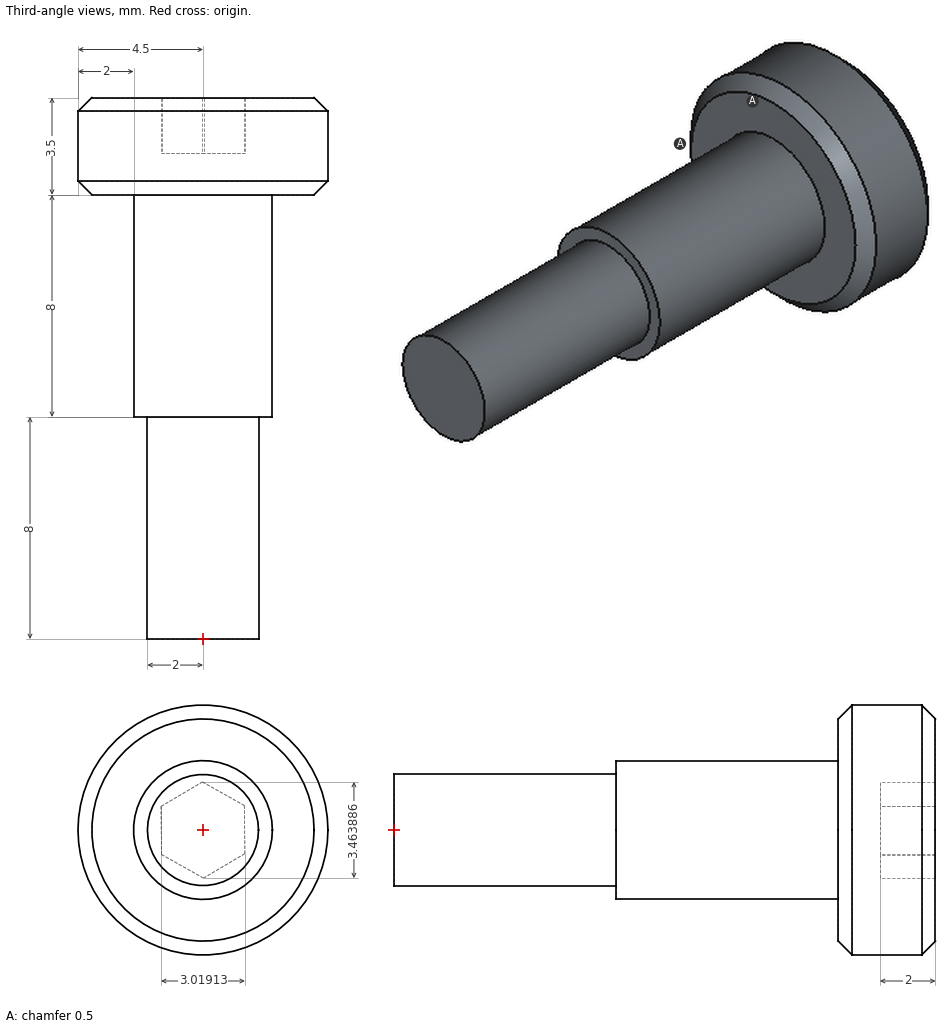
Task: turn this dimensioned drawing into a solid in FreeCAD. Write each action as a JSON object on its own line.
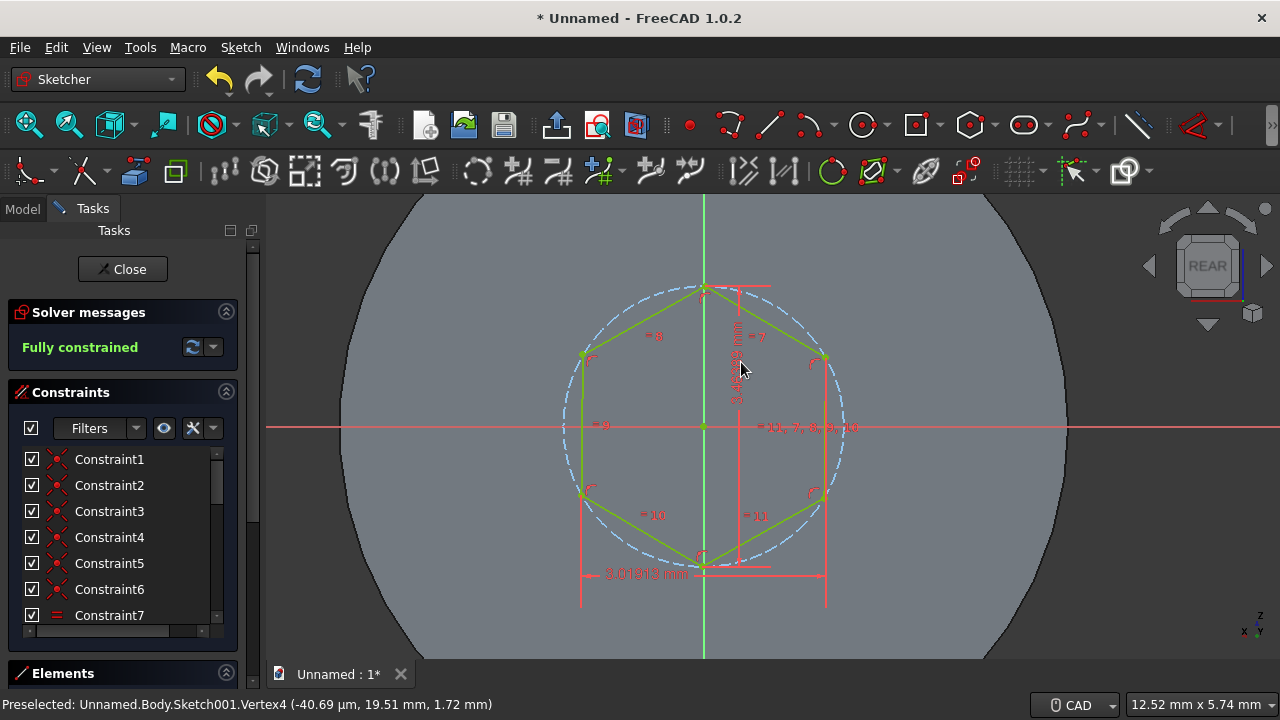
{"action": "left_click", "coordinate": [123, 269]}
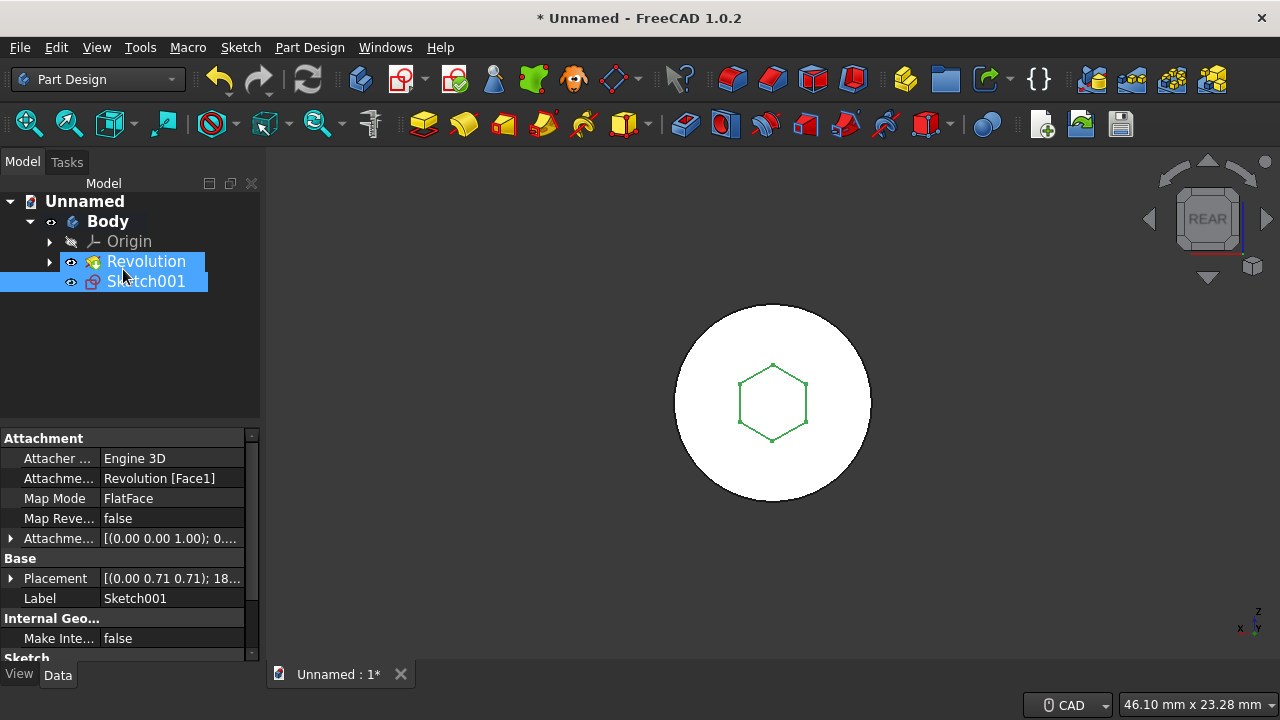
{"action": "left_click", "coordinate": [686, 124]}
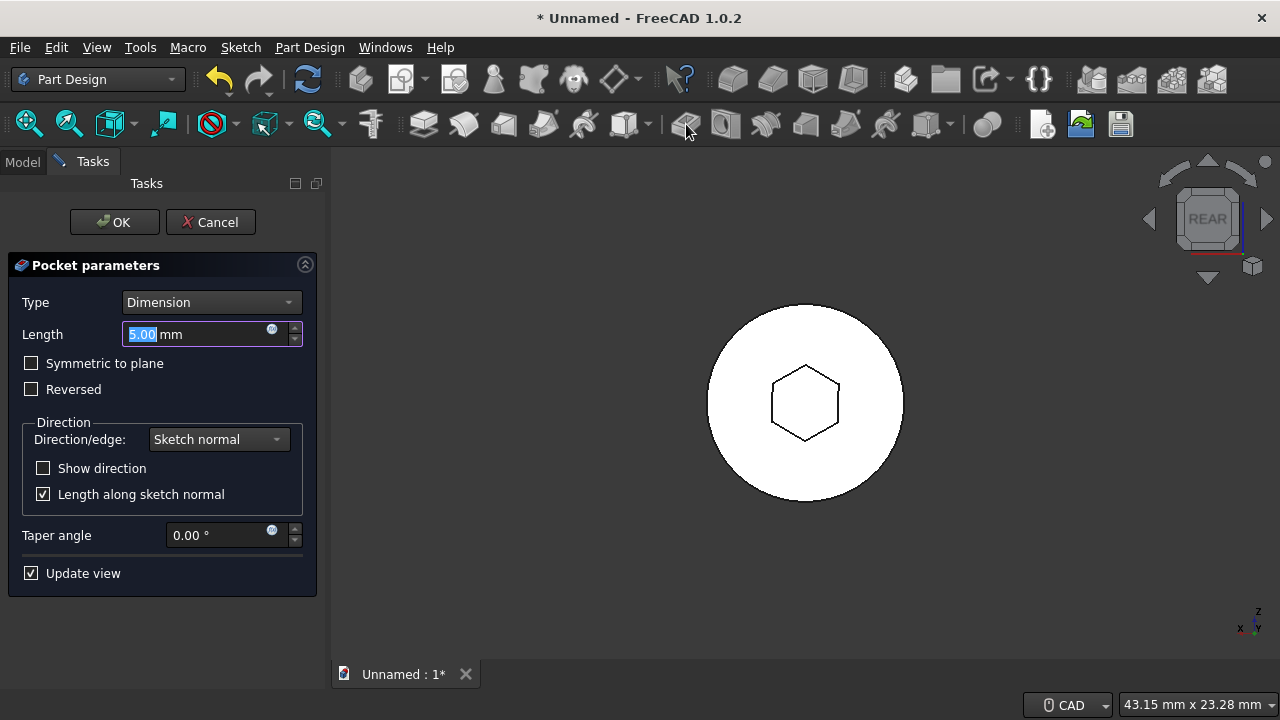
{"action": "type", "text": "2"}
{"action": "key", "text": "Tab"}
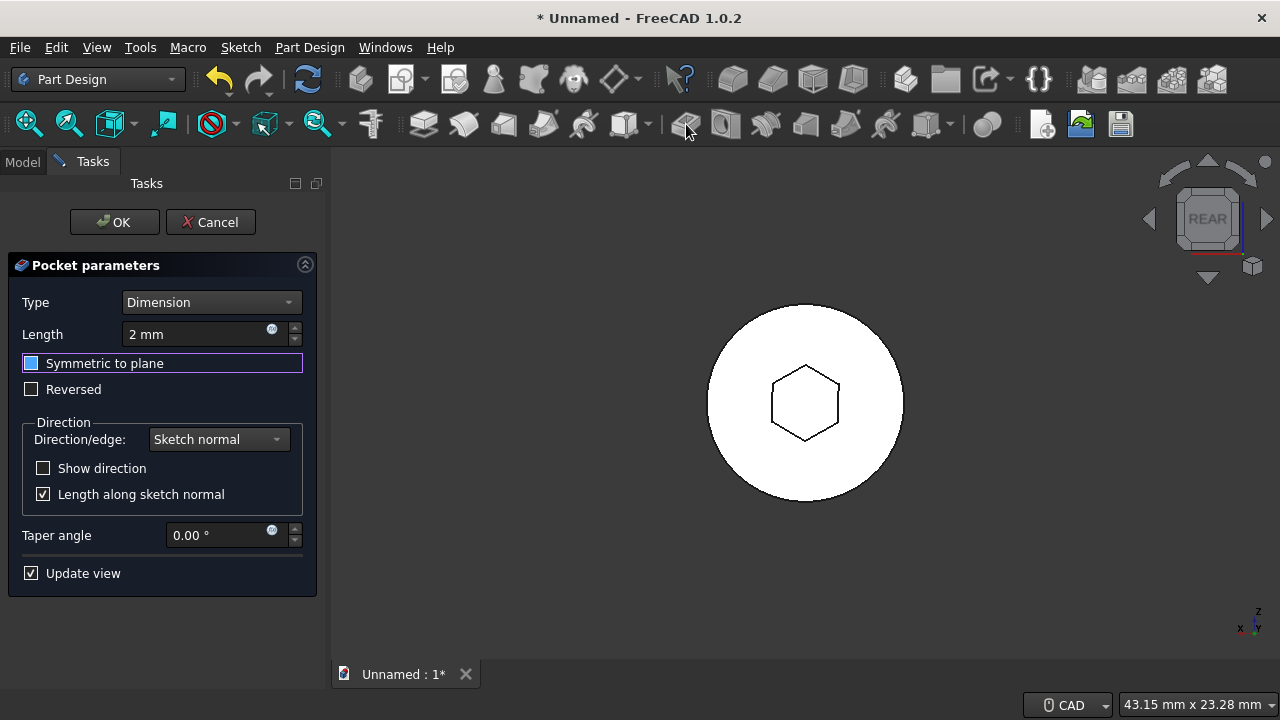
{"action": "left_click", "coordinate": [115, 222]}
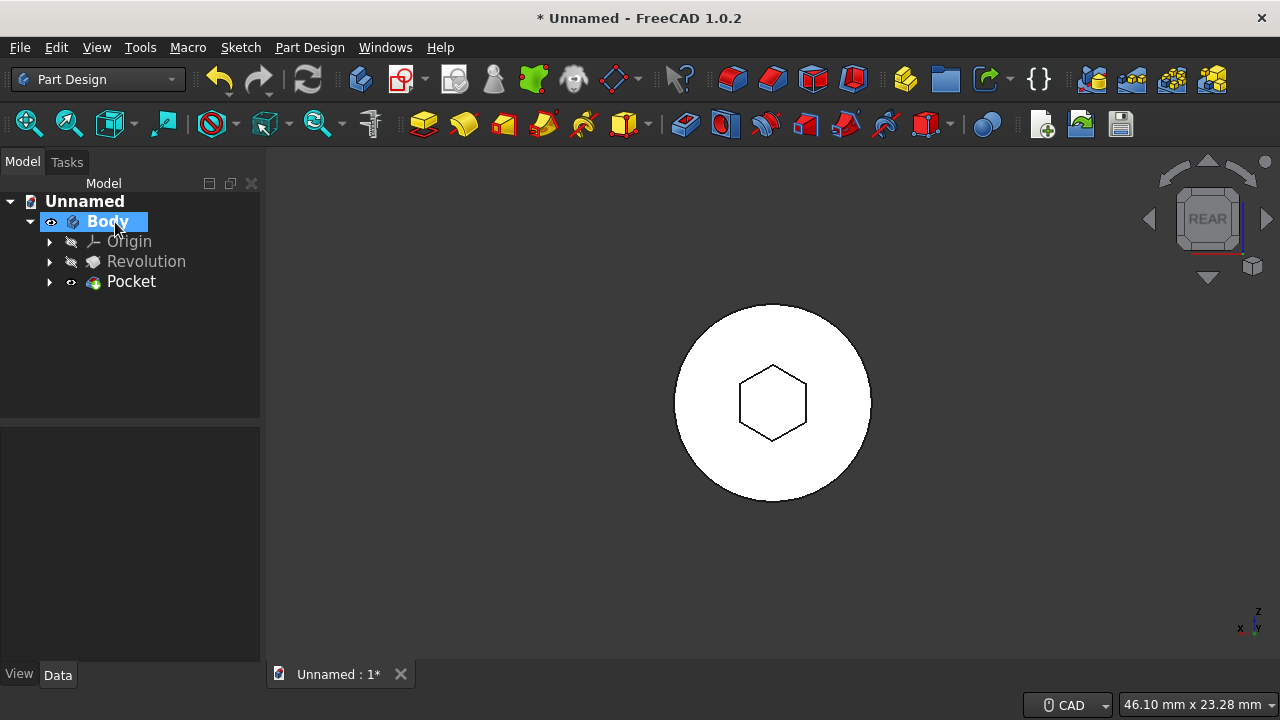
{"action": "left_click", "coordinate": [30, 124]}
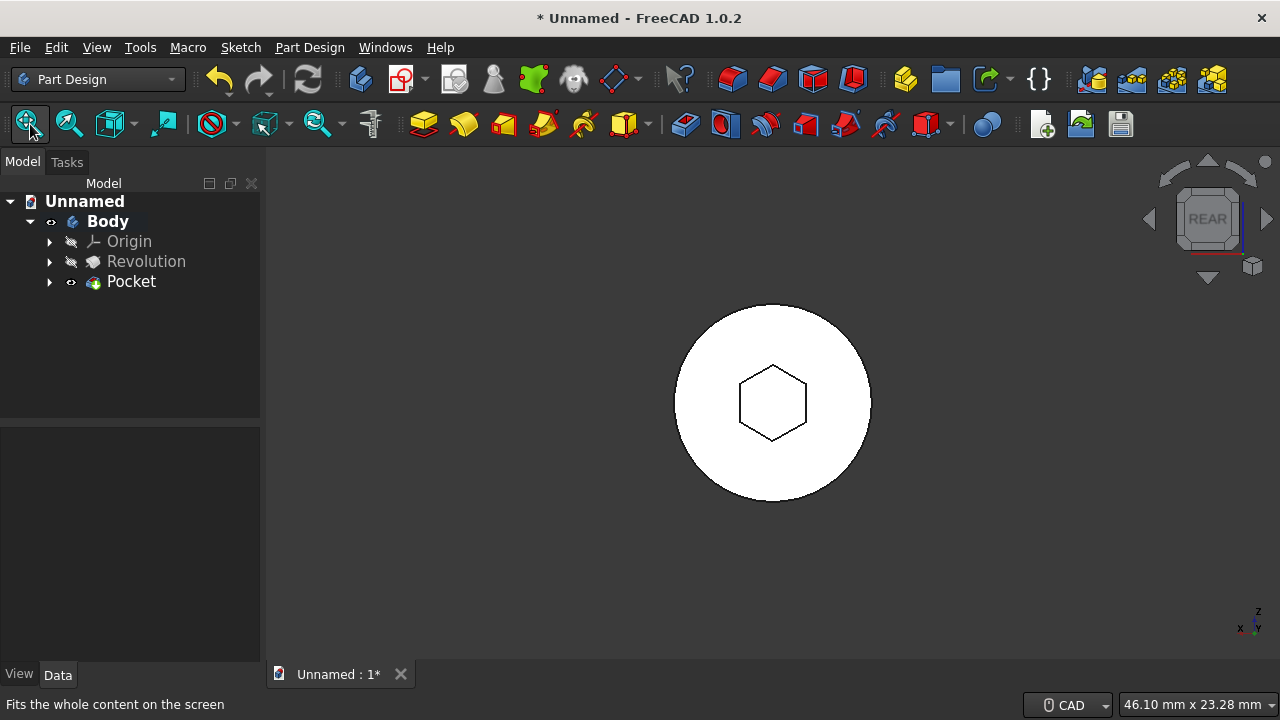
{"action": "left_click", "coordinate": [693, 344]}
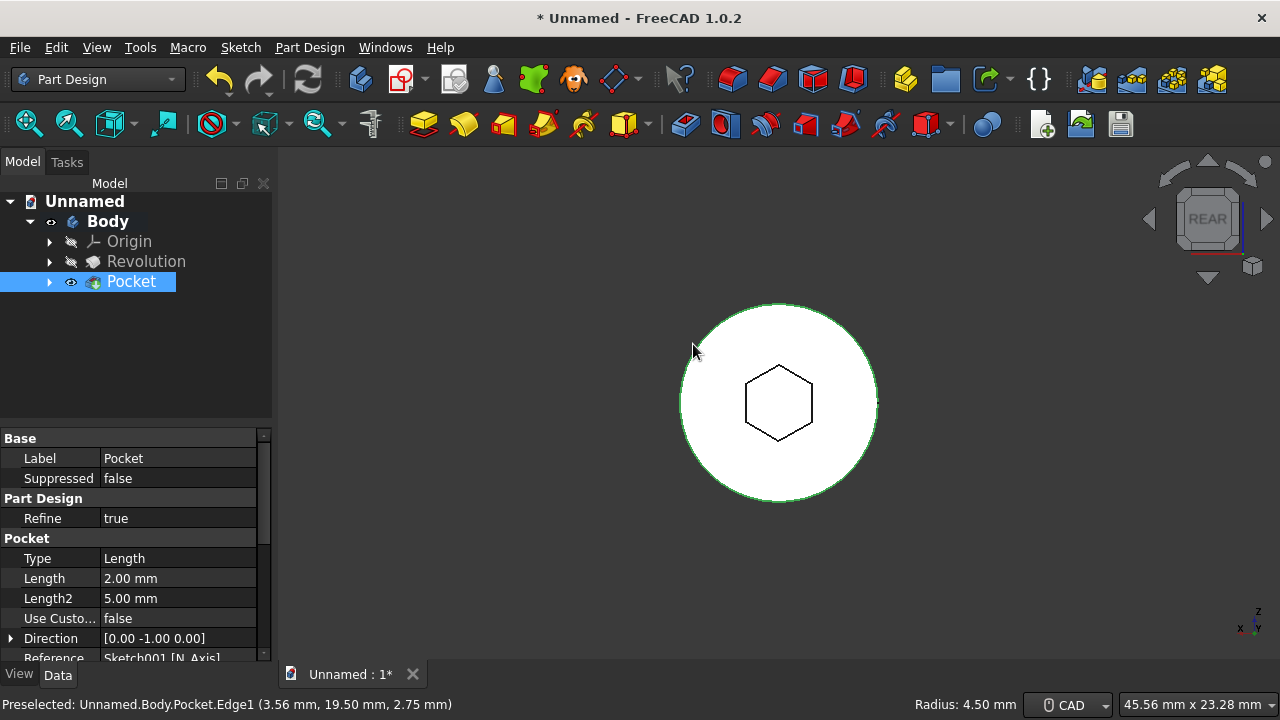
{"action": "key", "text": "0"}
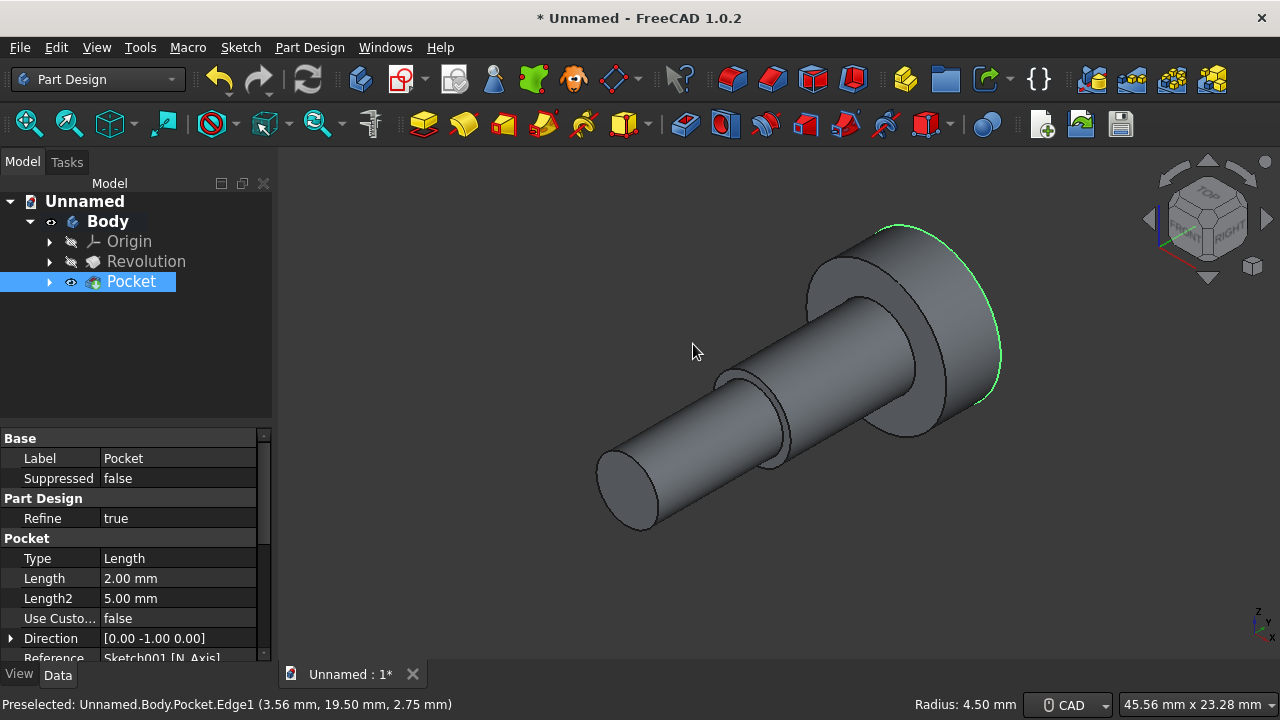
{"action": "left_click", "coordinate": [946, 386], "text": "ctrl"}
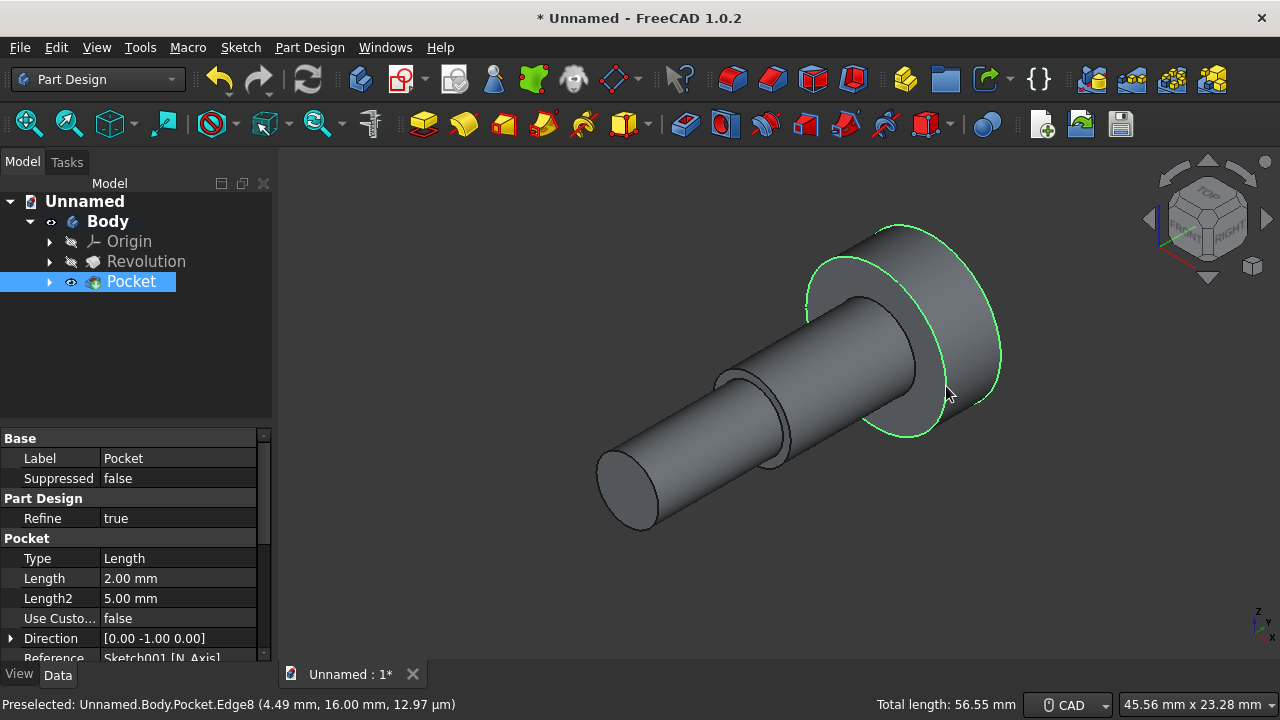
{"action": "left_click", "coordinate": [774, 80]}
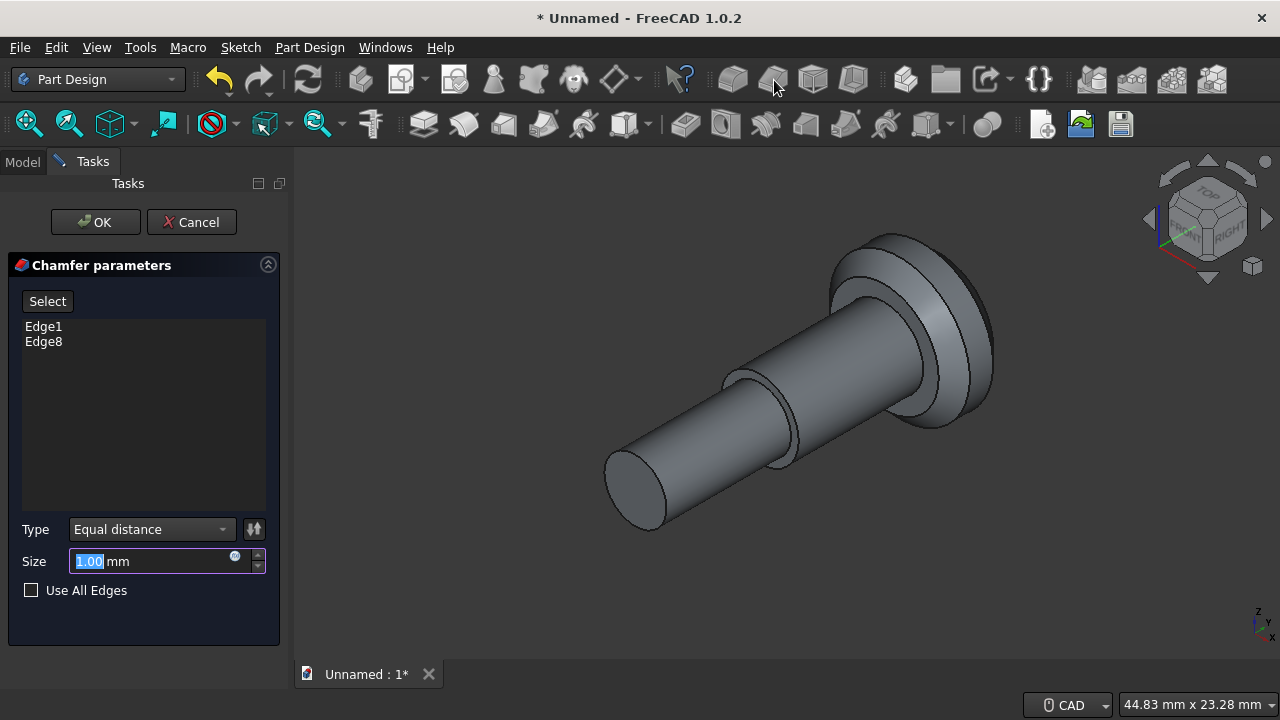
{"action": "type", "text": "0.5"}
{"action": "key", "text": "Tab"}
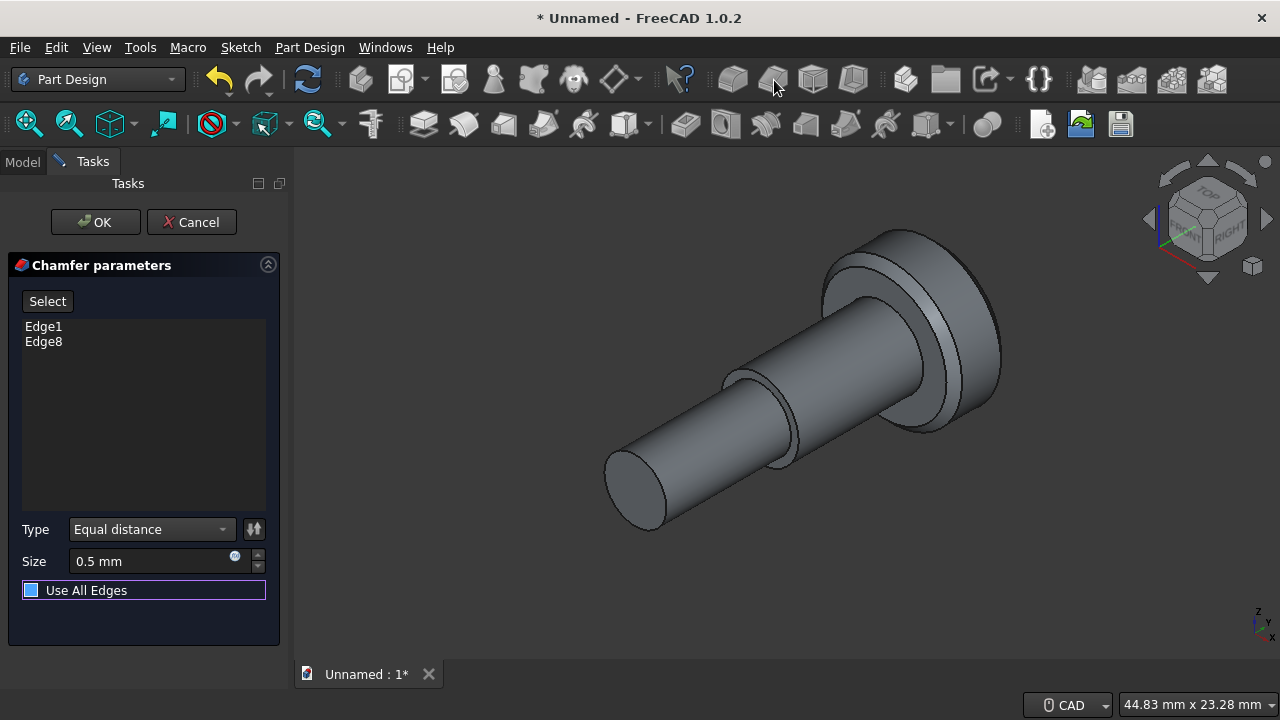
{"action": "left_click", "coordinate": [96, 222]}